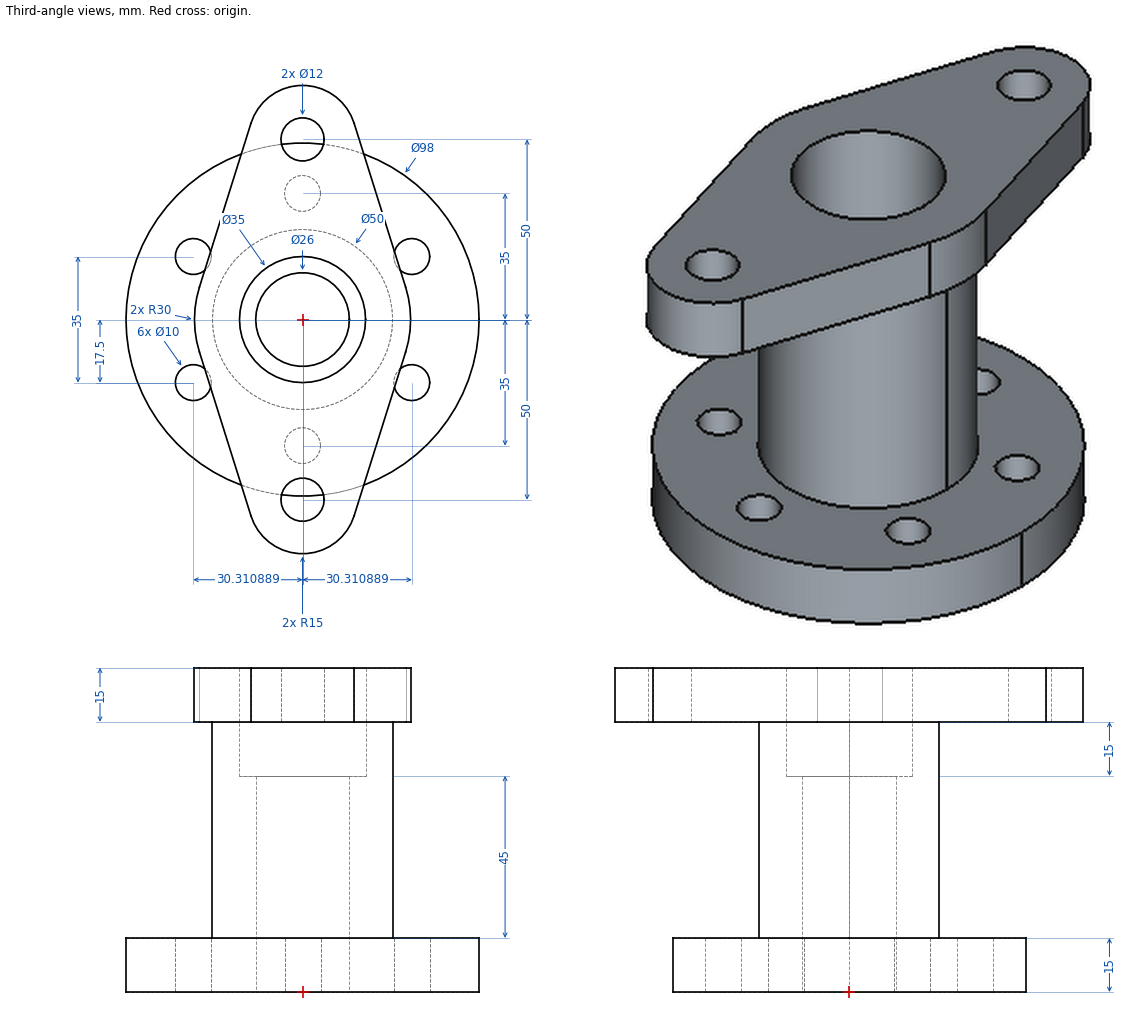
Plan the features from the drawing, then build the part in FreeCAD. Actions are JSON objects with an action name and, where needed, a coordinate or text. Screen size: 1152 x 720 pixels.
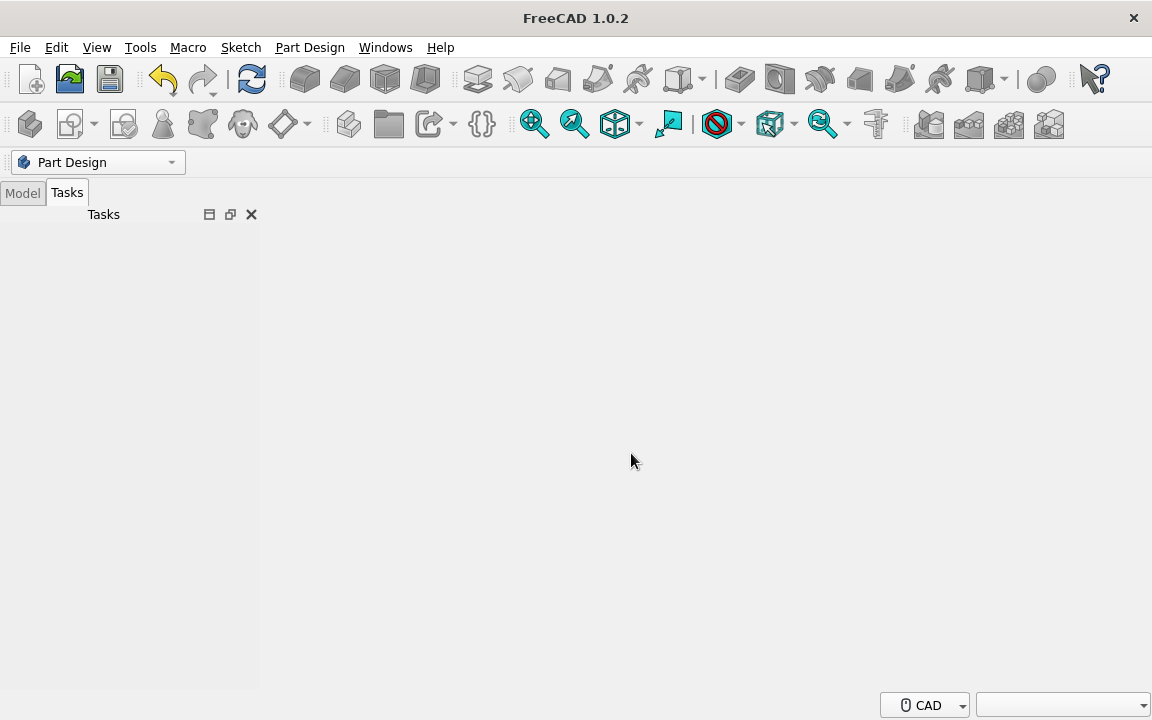
{"action": "key", "text": "ctrl+n"}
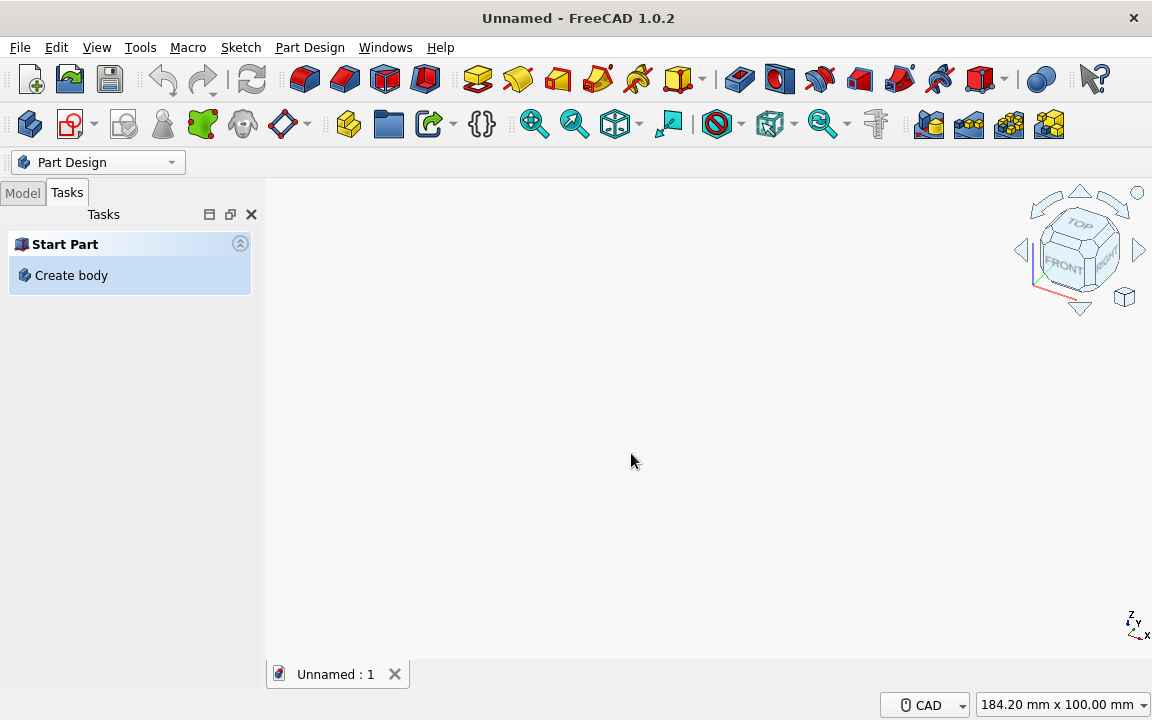
{"action": "left_click", "coordinate": [70, 124]}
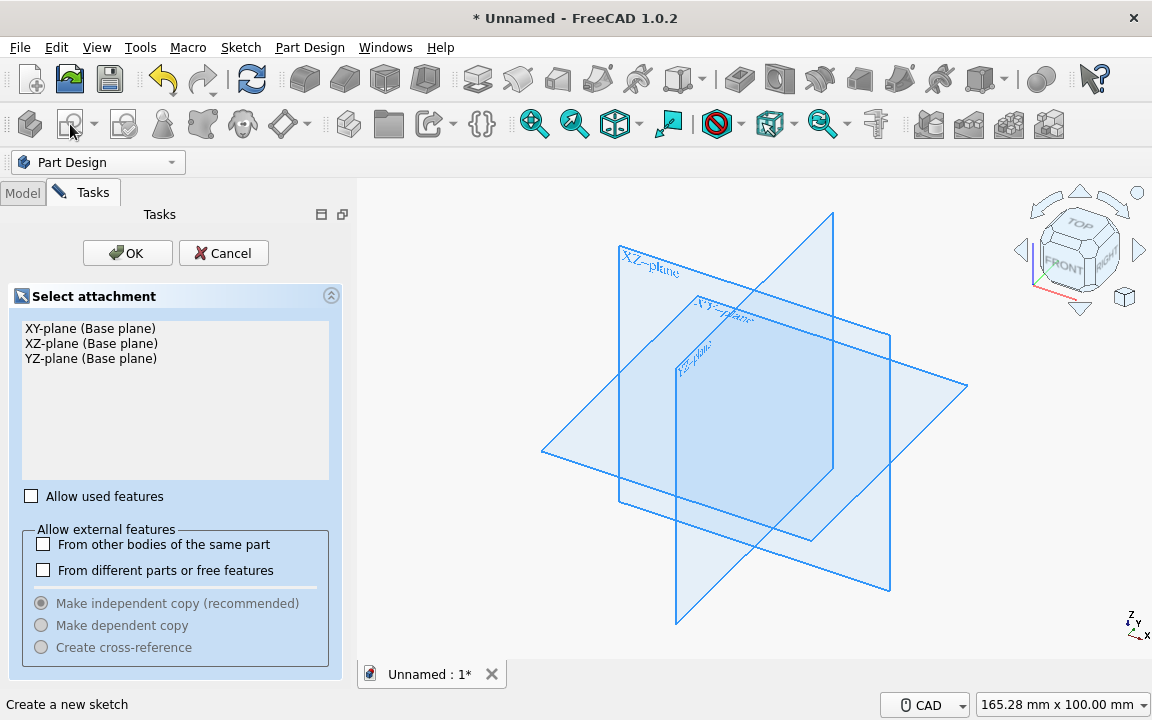
{"action": "left_click", "coordinate": [82, 328]}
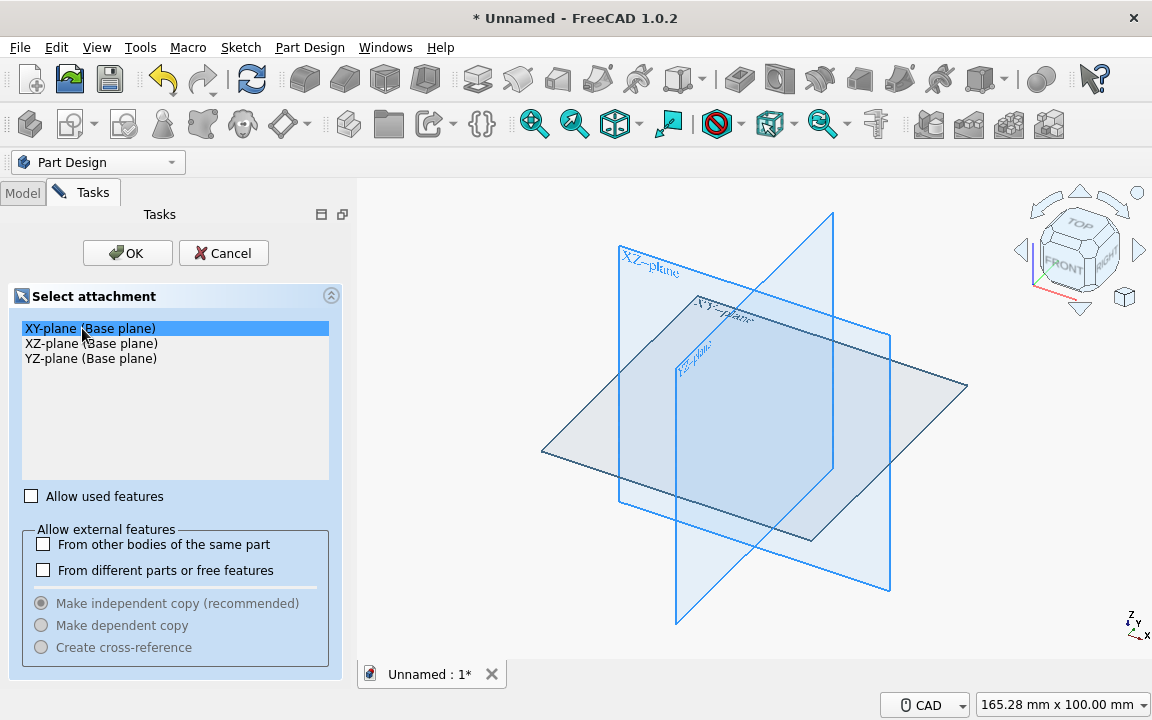
{"action": "left_click", "coordinate": [128, 253]}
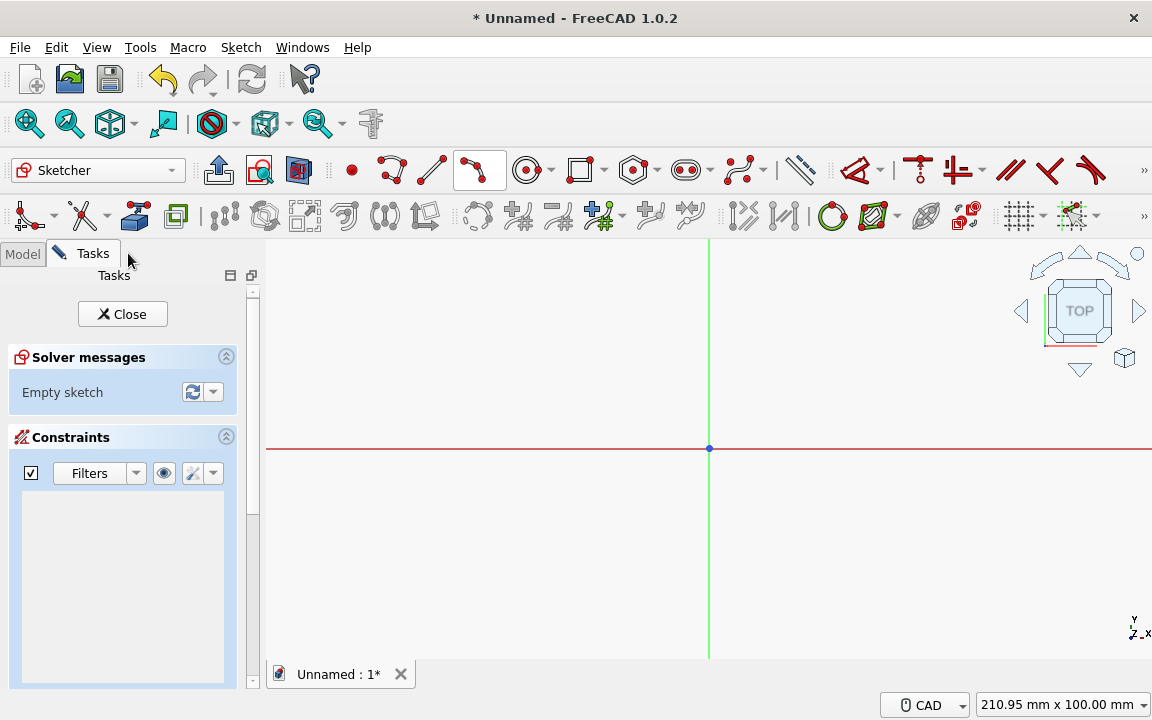
{"action": "scroll", "coordinate": [501, 449], "scroll_direction": "down", "scroll_amount": 2}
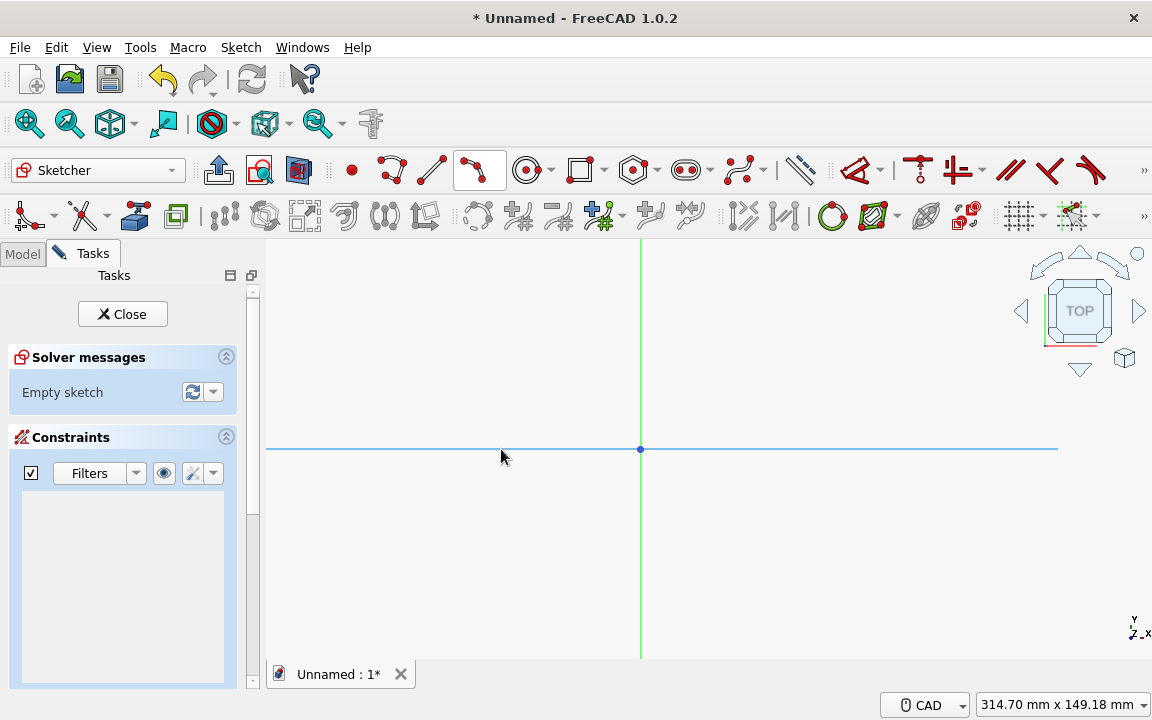
{"action": "key", "text": "g c"}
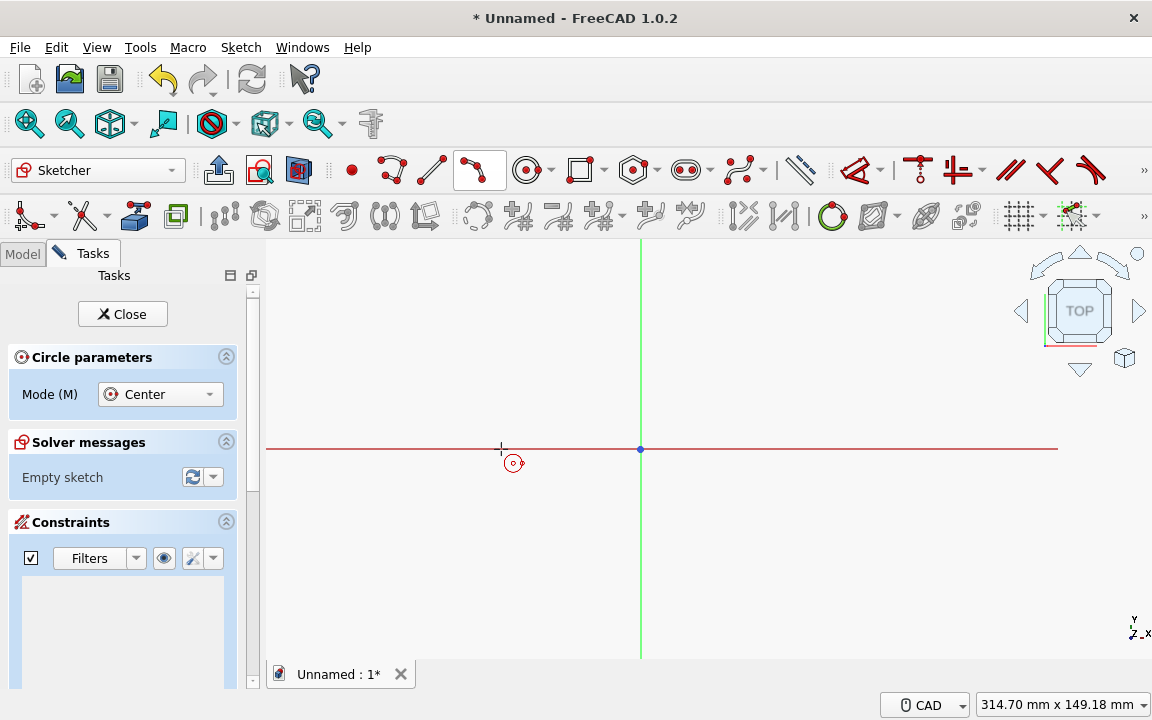
{"action": "left_click", "coordinate": [641, 449]}
{"action": "left_click", "coordinate": [738, 352]}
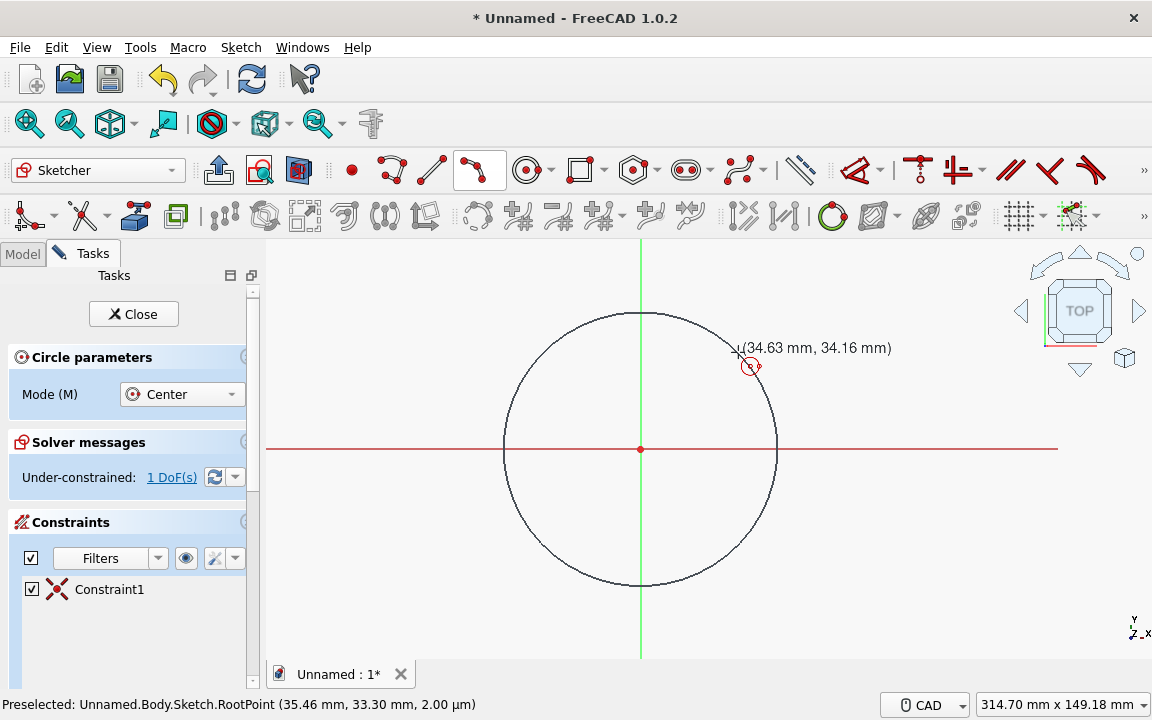
{"action": "scroll", "coordinate": [555, 498], "scroll_direction": "up", "scroll_amount": 3}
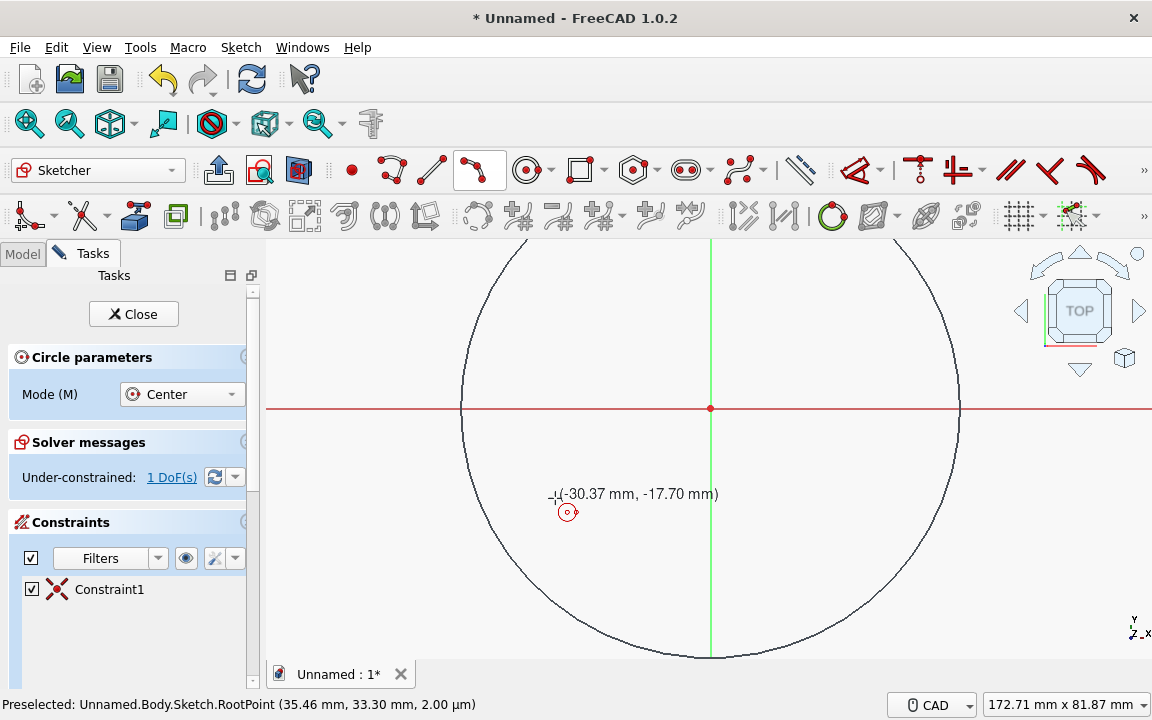
{"action": "left_click", "coordinate": [555, 498]}
{"action": "left_click", "coordinate": [573, 480]}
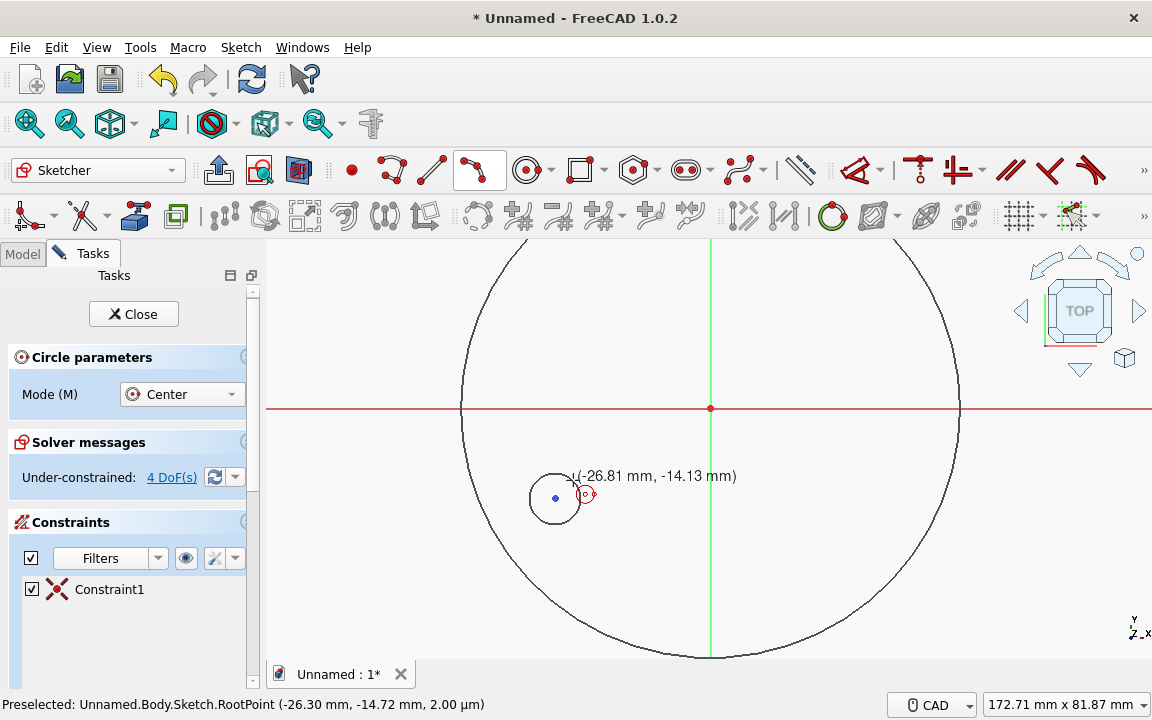
{"action": "left_click", "coordinate": [711, 588]}
{"action": "left_click", "coordinate": [729, 570]}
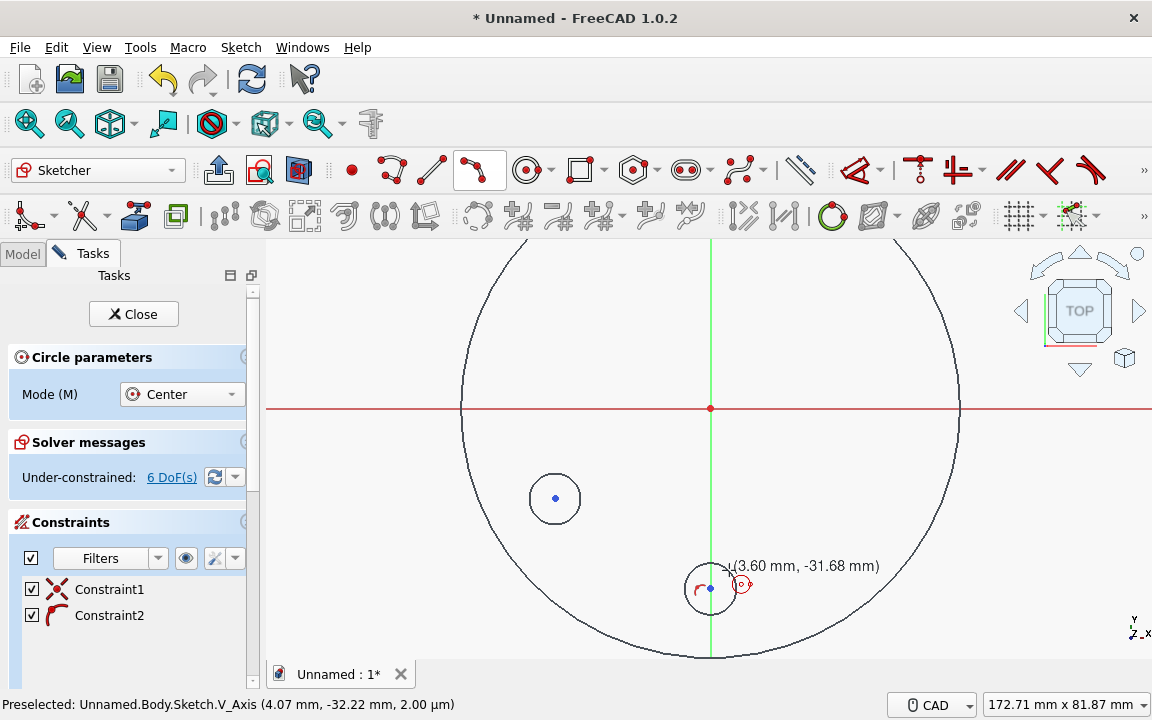
{"action": "left_click", "coordinate": [866, 498]}
{"action": "left_click", "coordinate": [884, 480]}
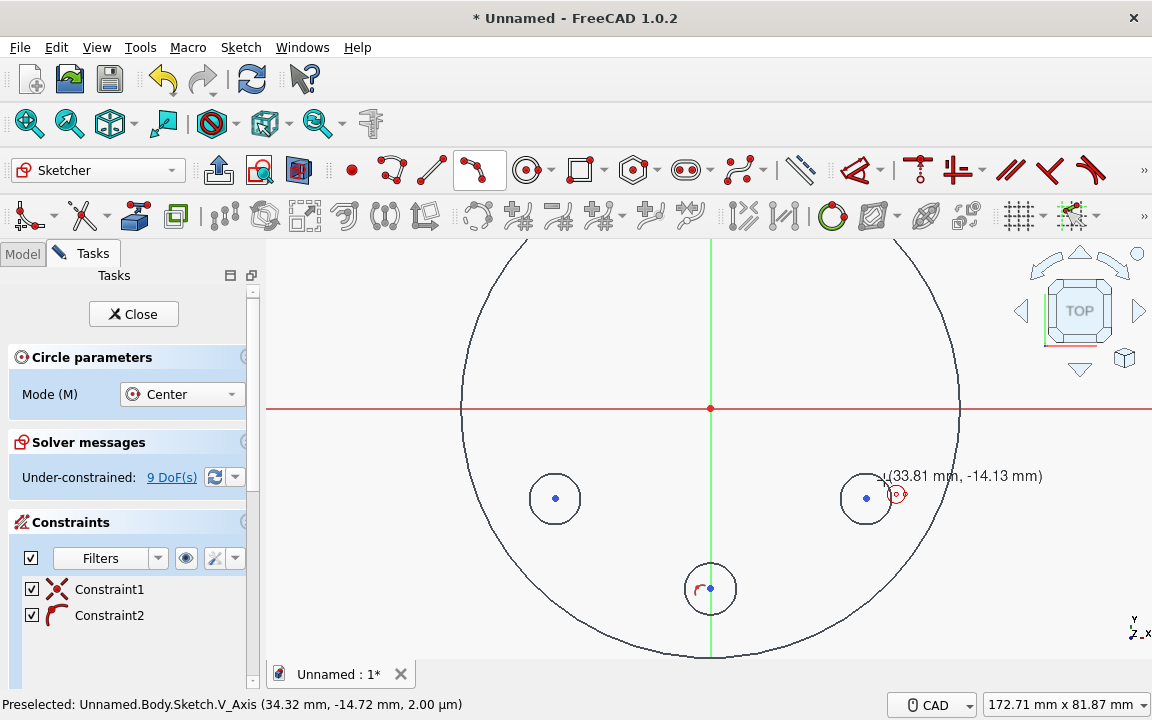
{"action": "left_click", "coordinate": [555, 319]}
{"action": "left_click", "coordinate": [573, 301]}